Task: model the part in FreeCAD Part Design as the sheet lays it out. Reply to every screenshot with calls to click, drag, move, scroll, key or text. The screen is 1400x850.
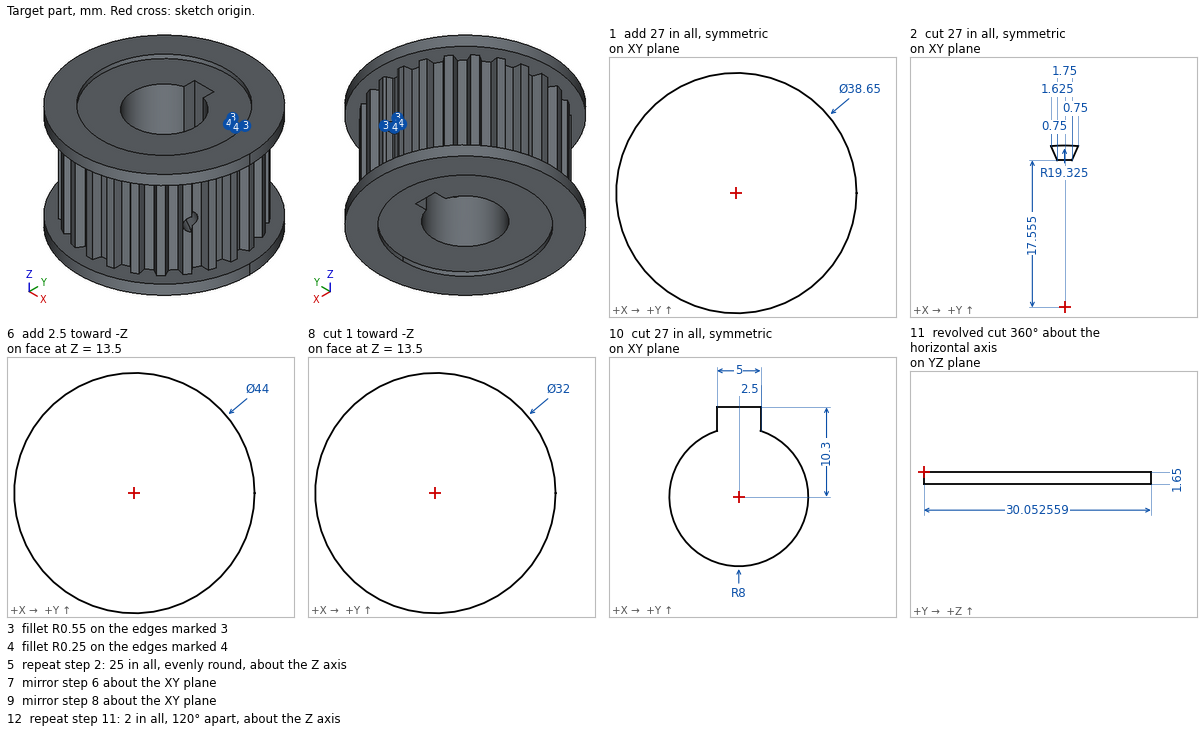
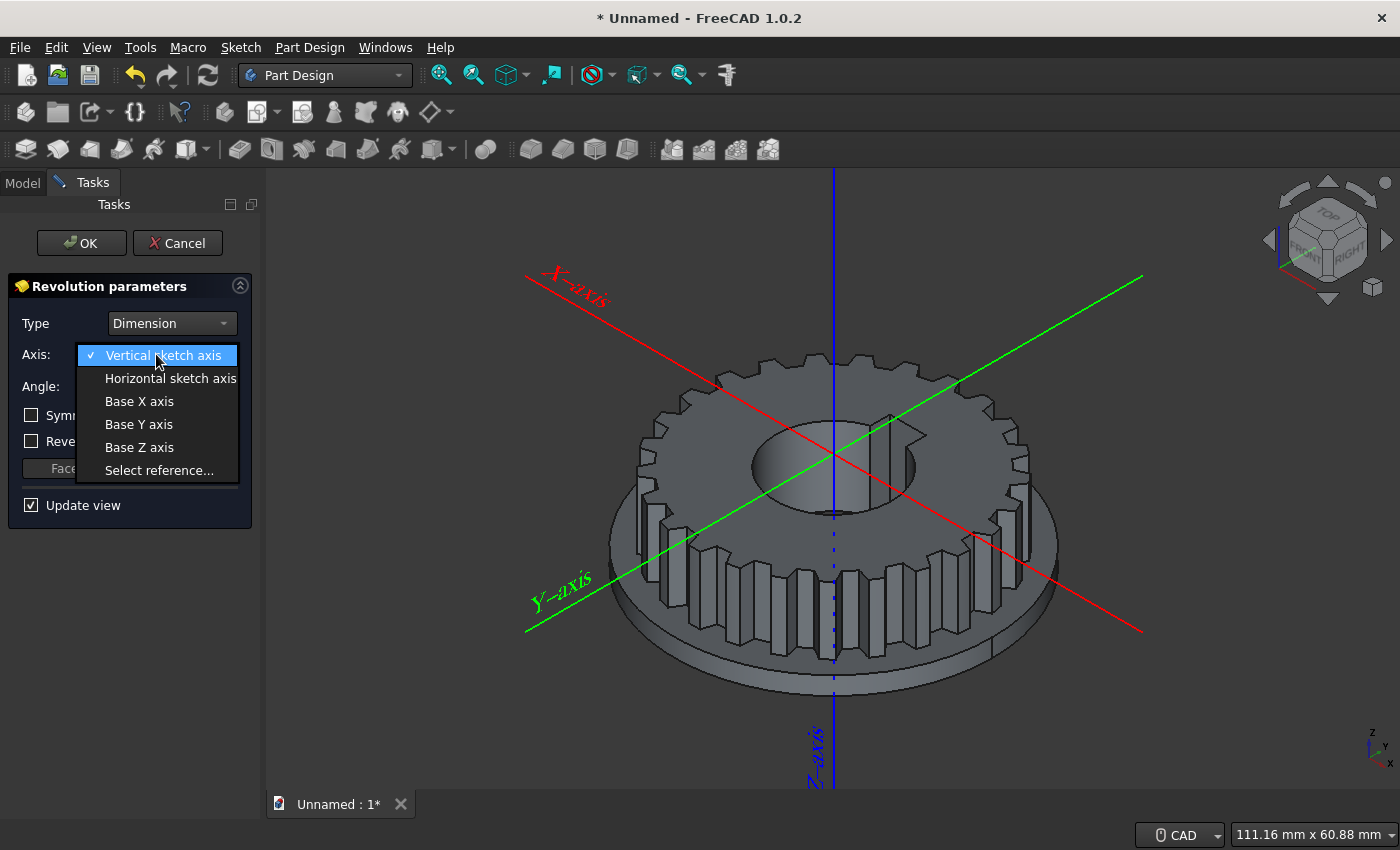
click(156, 378)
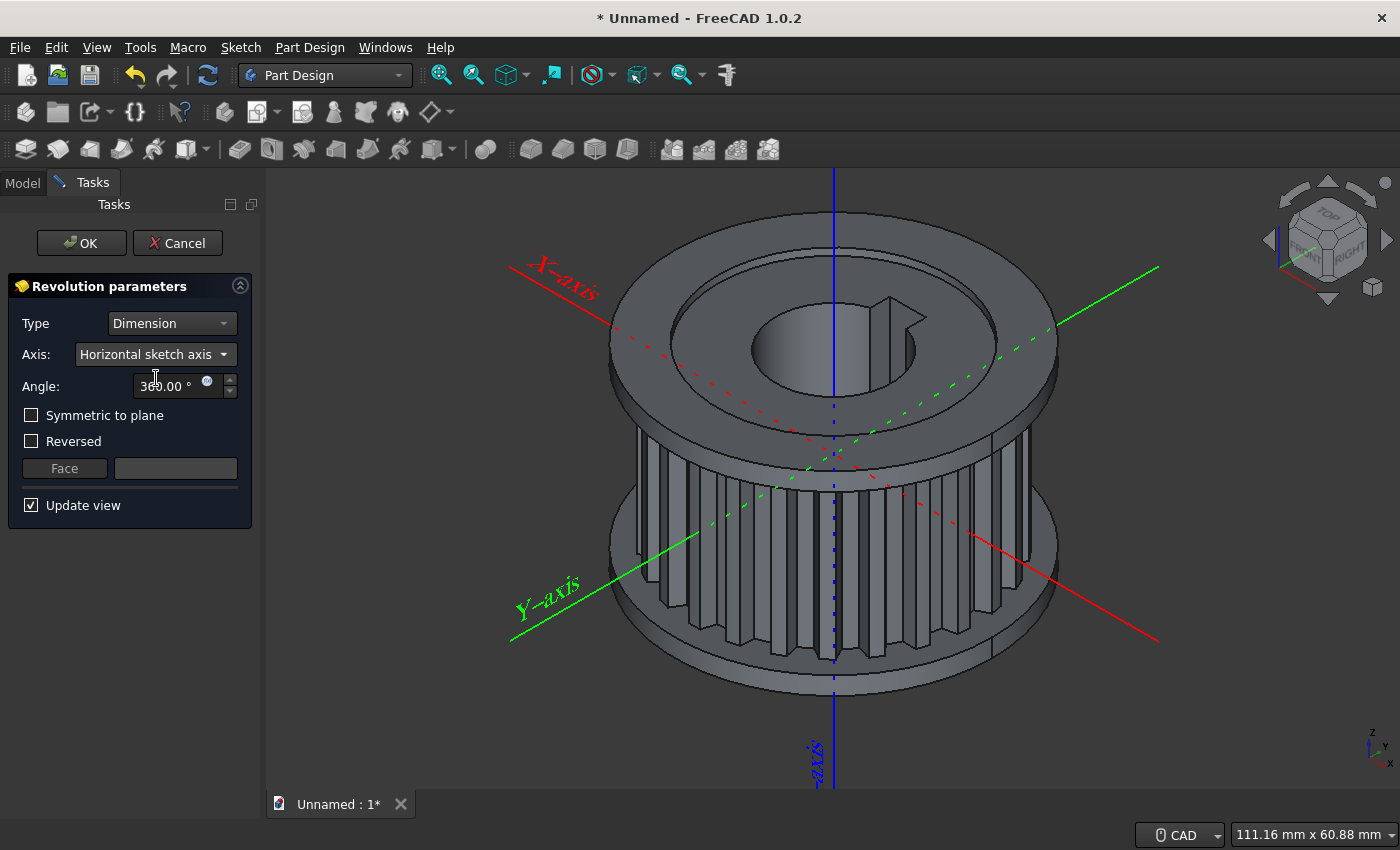
click(82, 243)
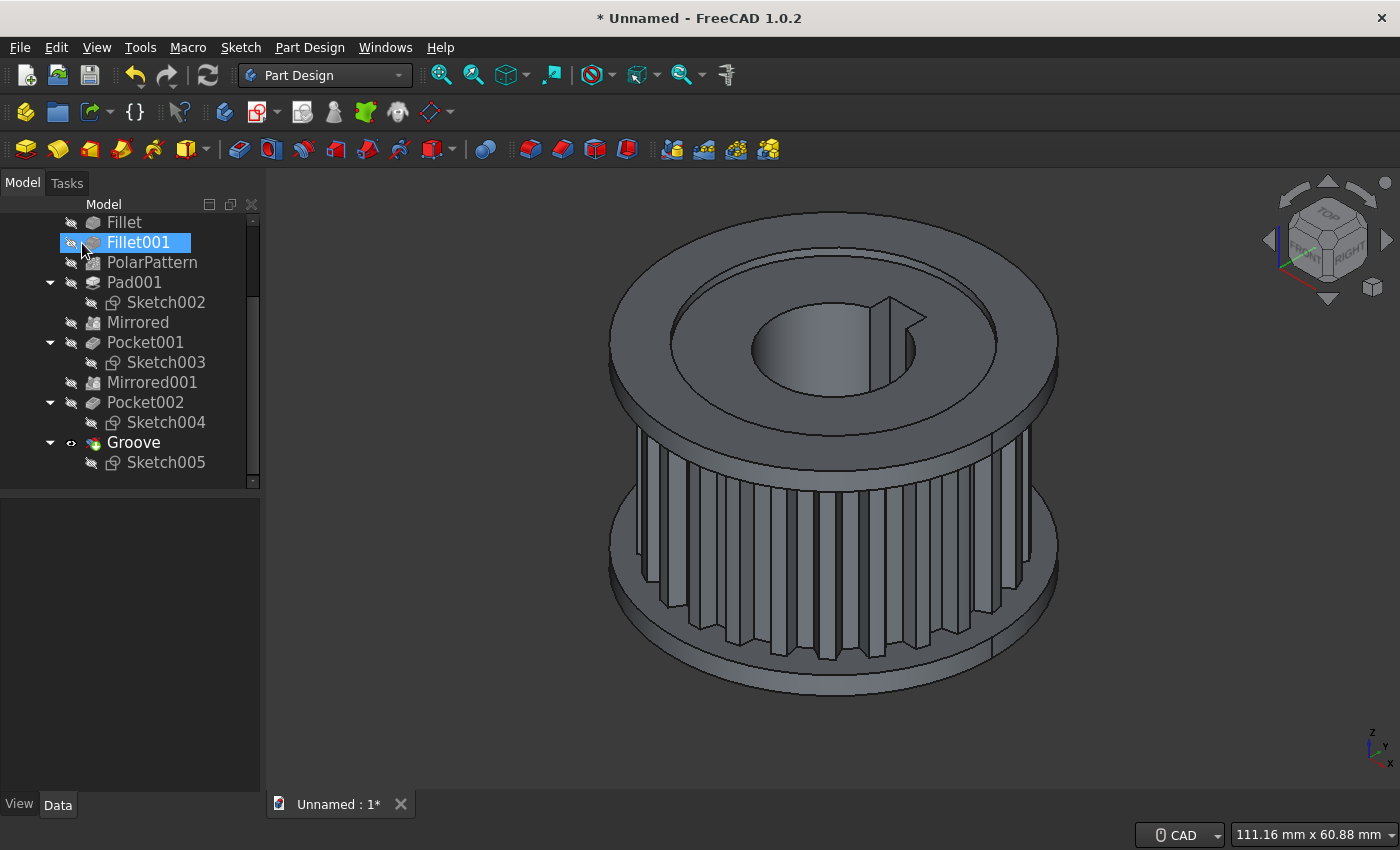
click(442, 76)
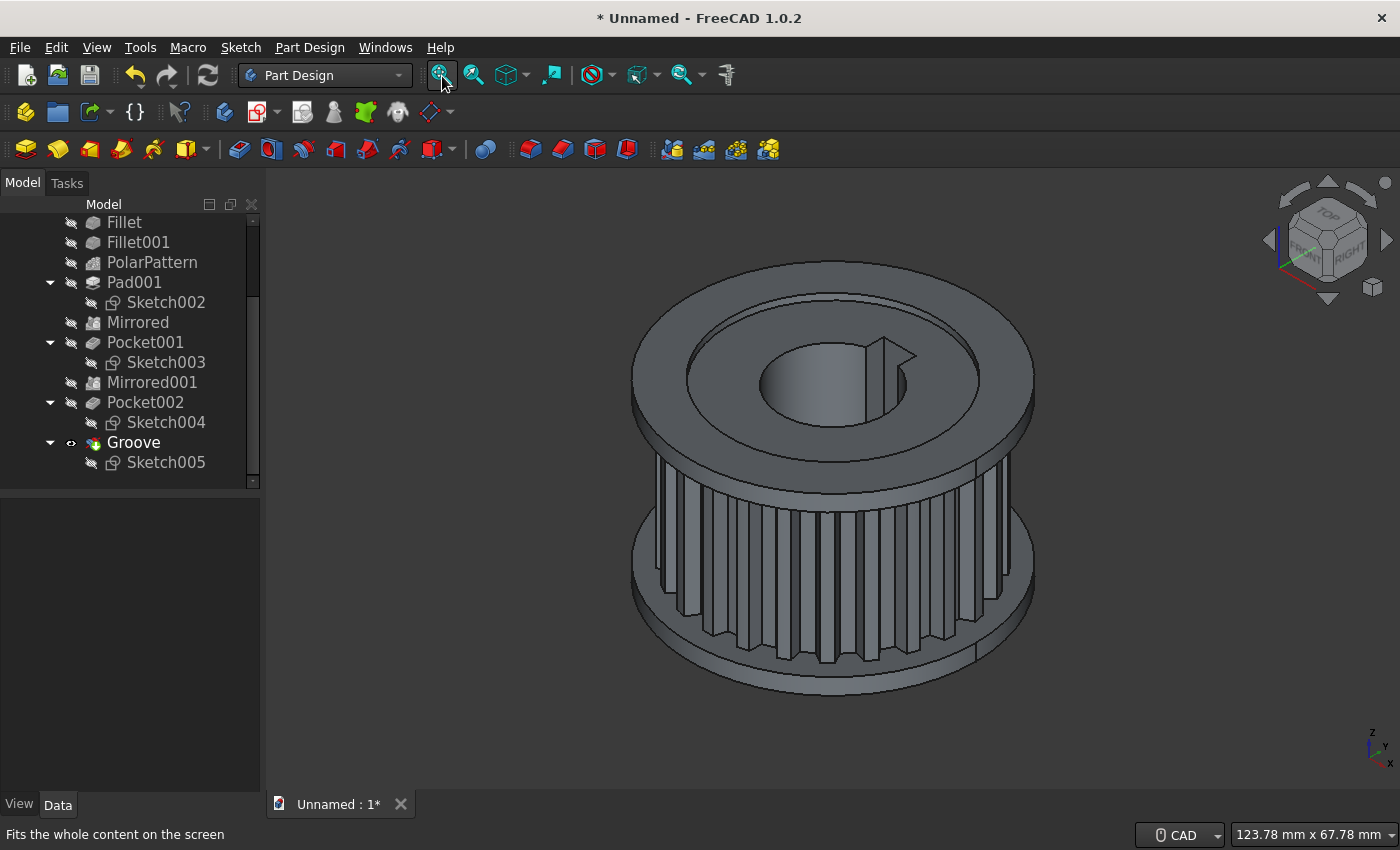
click(116, 443)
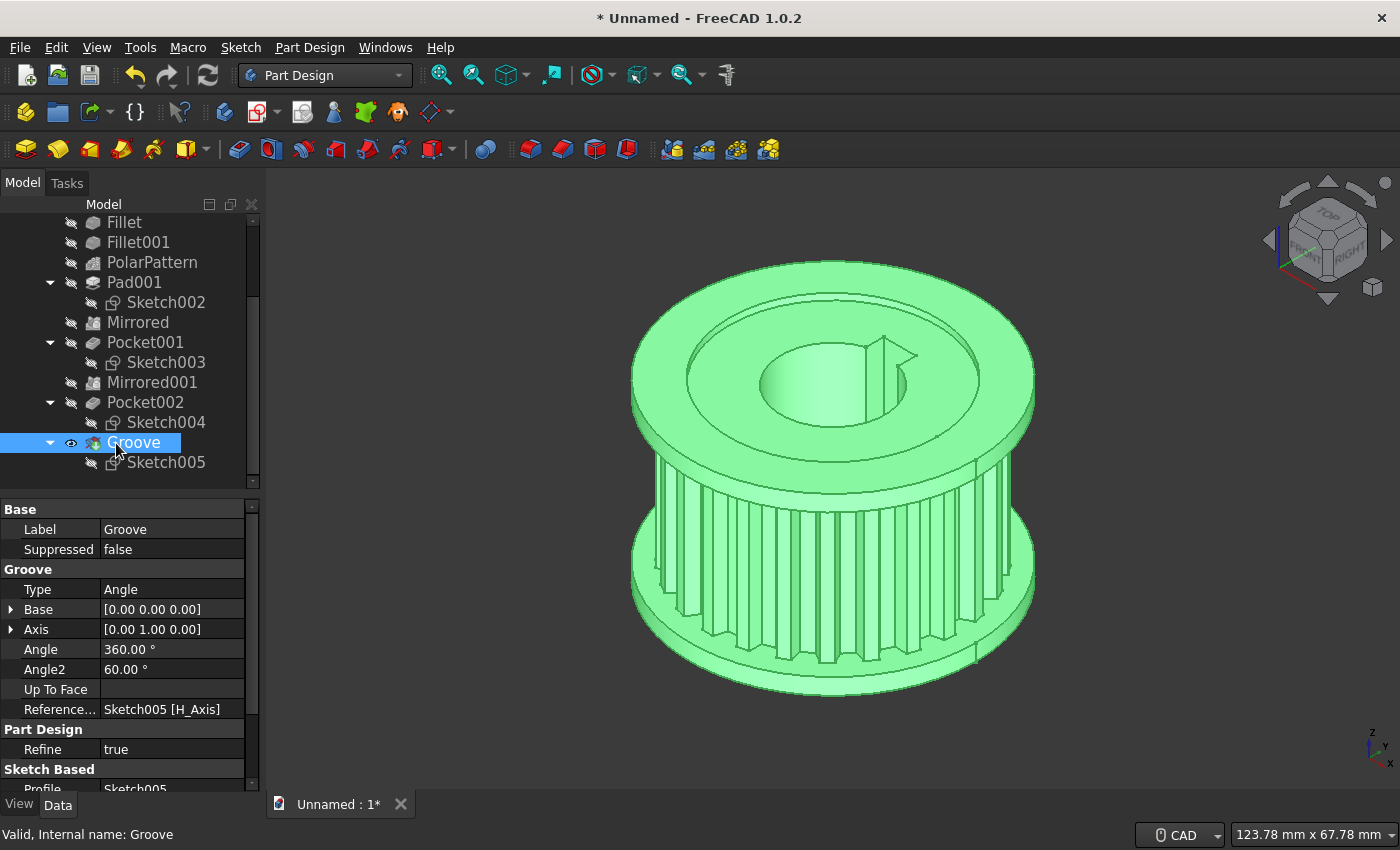
click(736, 150)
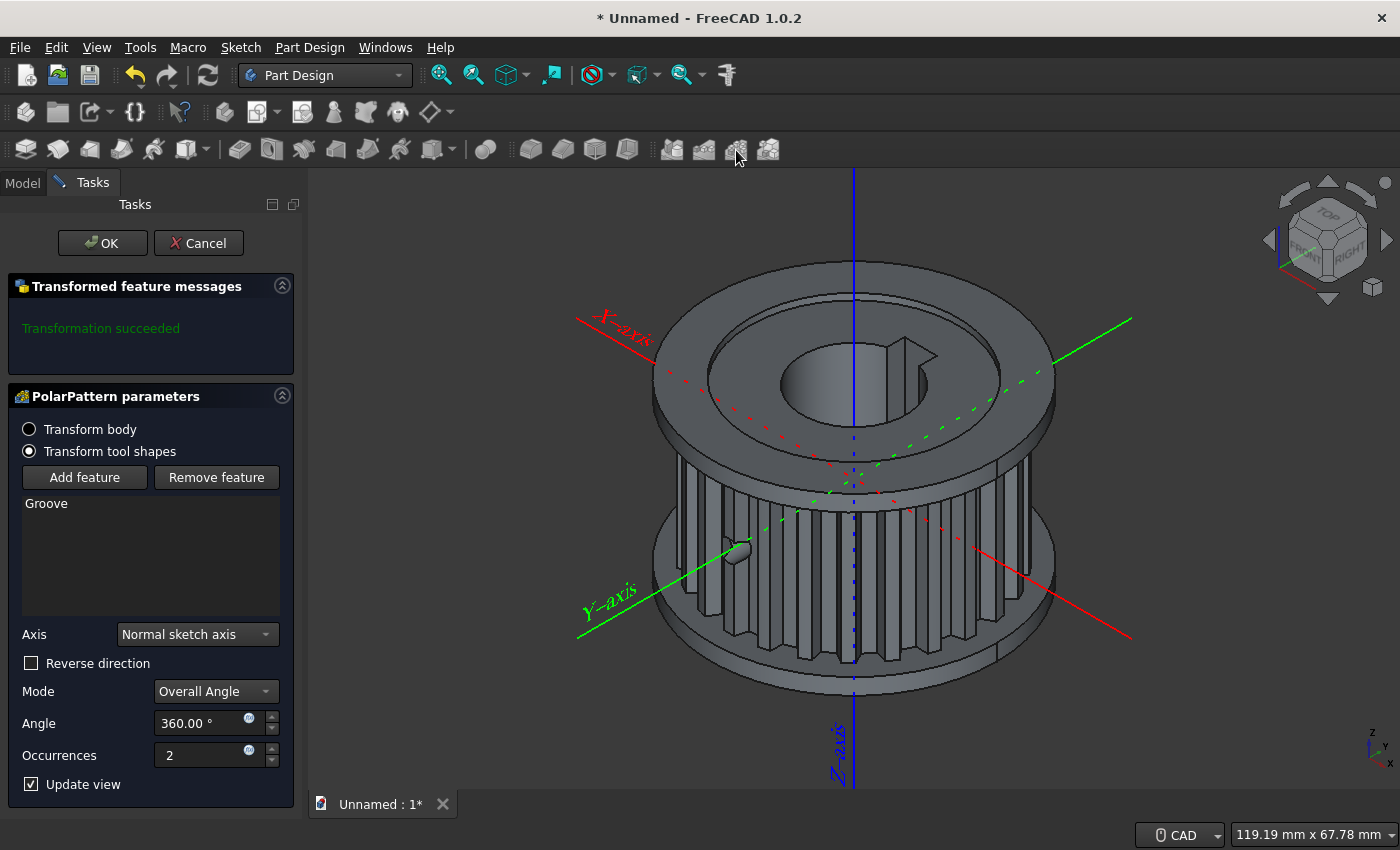
click(198, 634)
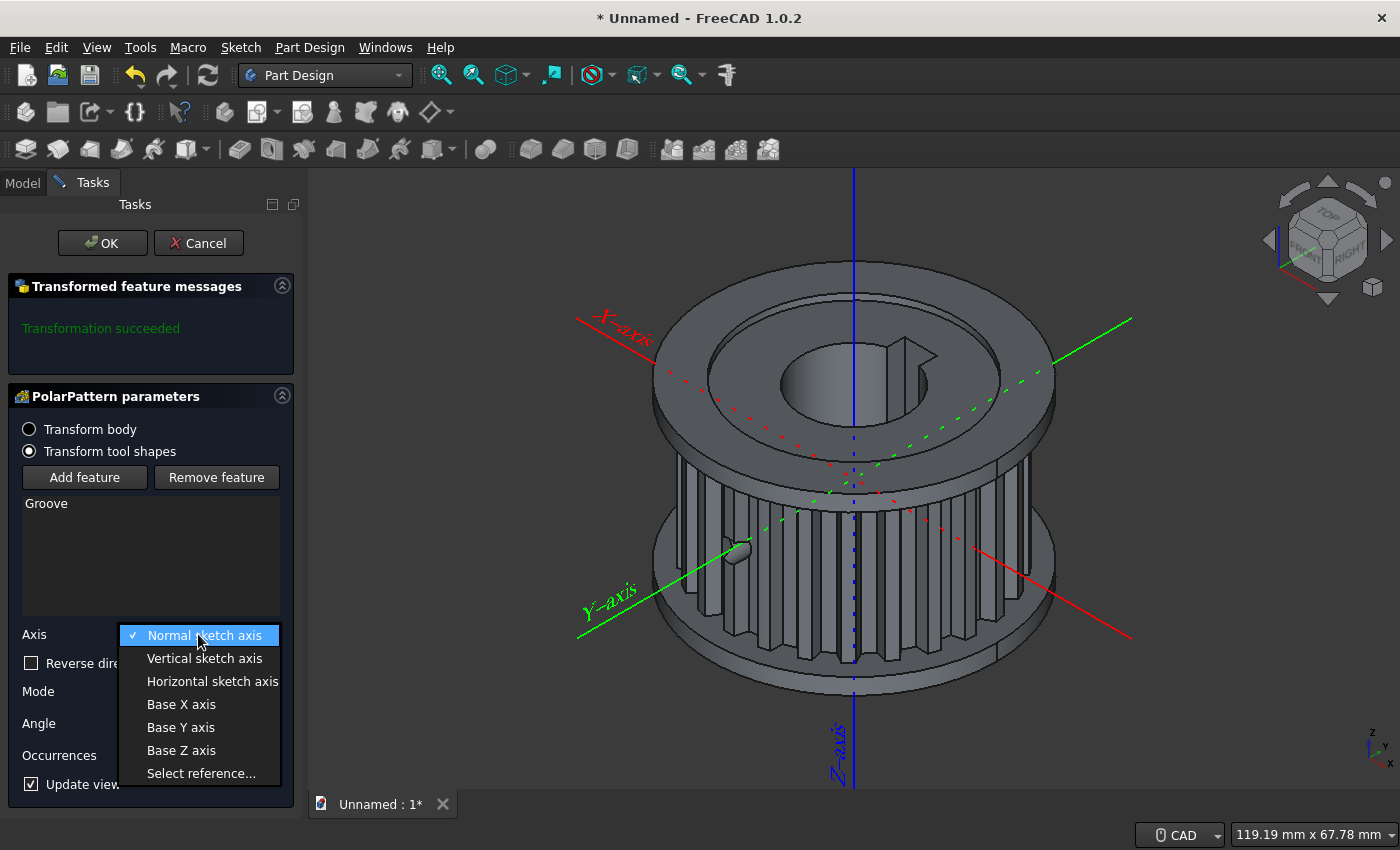
click(198, 750)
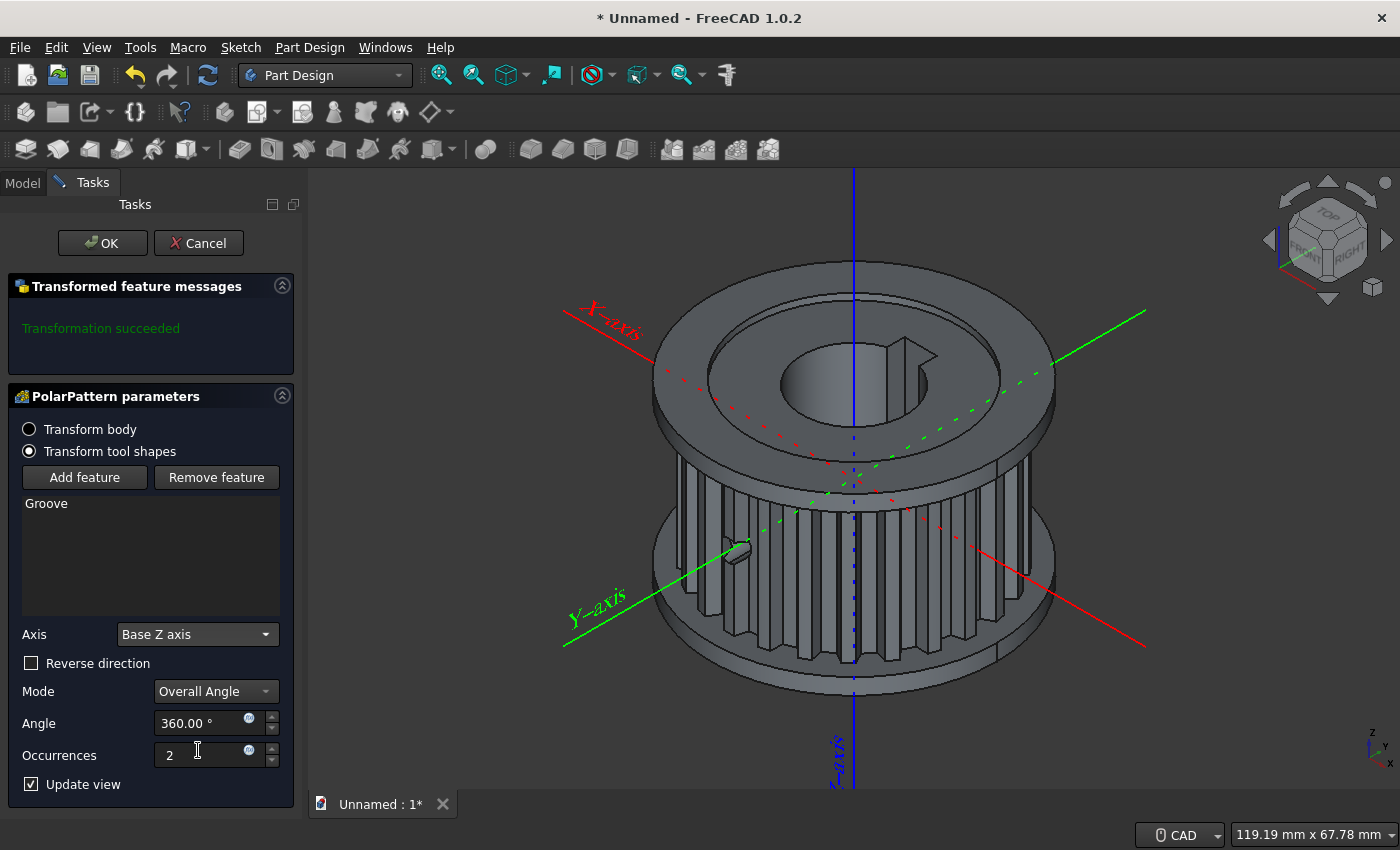
click(217, 692)